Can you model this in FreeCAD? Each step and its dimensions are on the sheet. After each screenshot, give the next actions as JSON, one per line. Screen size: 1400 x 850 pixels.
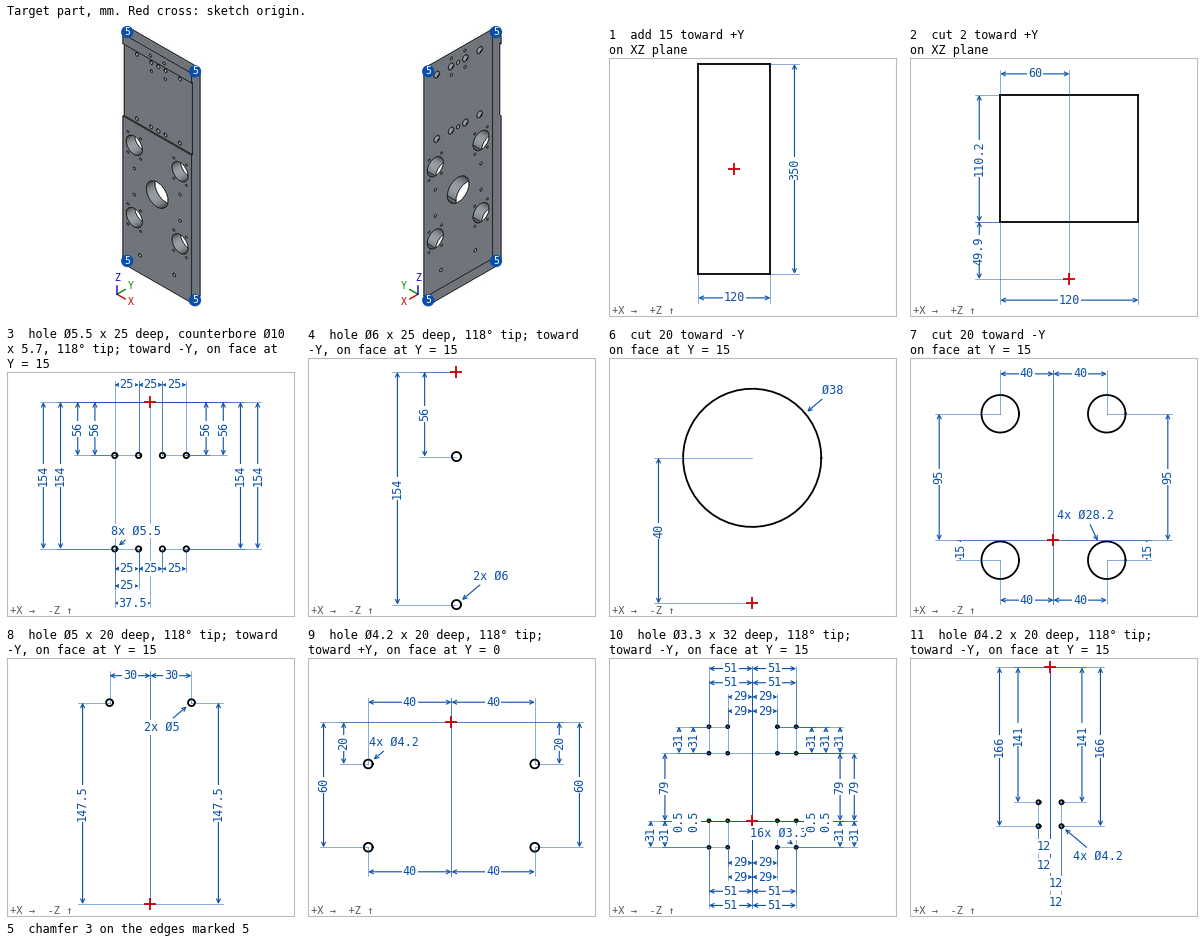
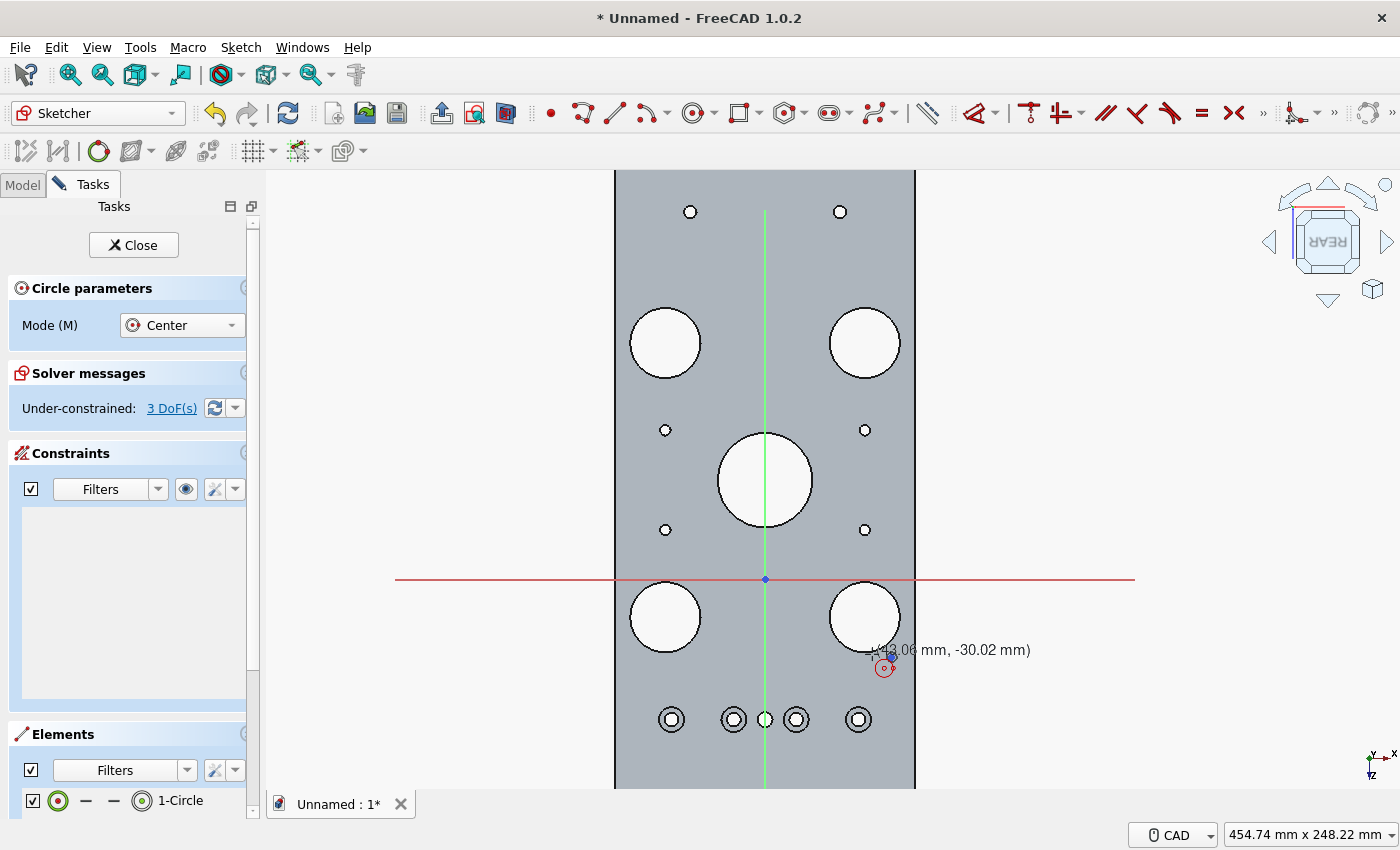
{"action": "left_click", "coordinate": [837, 656]}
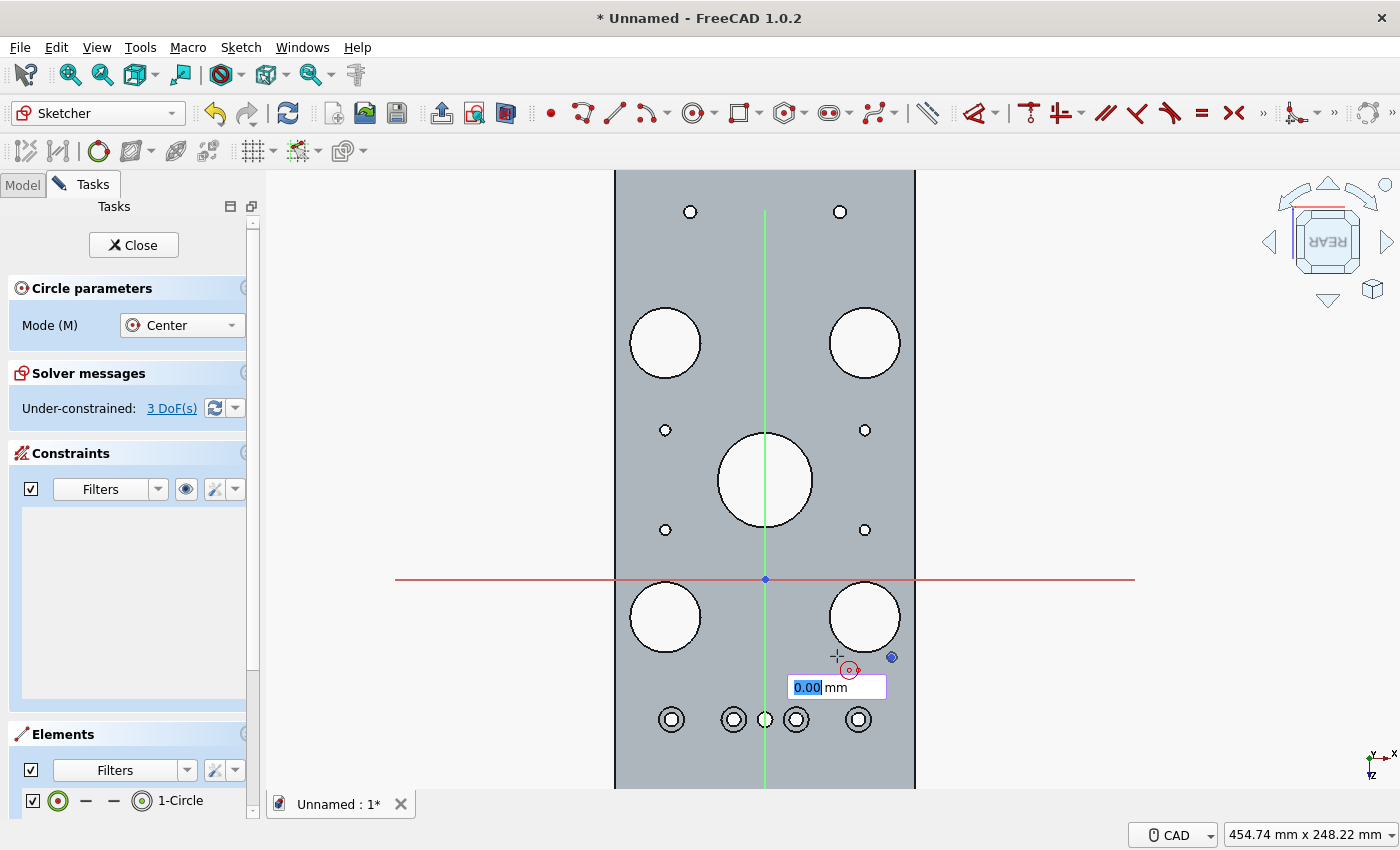
{"action": "scroll", "coordinate": [840, 653], "scroll_direction": "up", "scroll_amount": 7}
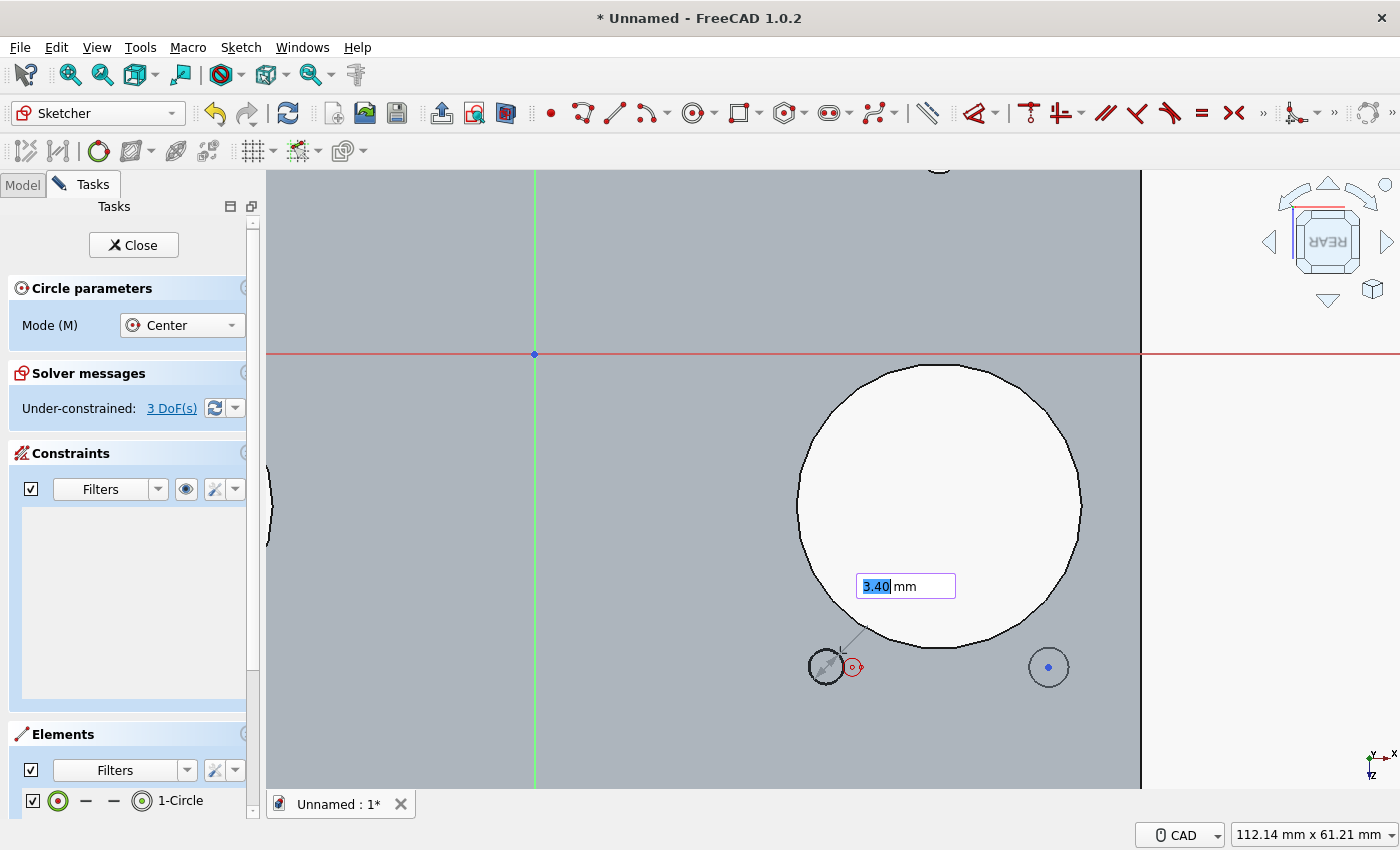
{"action": "left_click", "coordinate": [840, 651]}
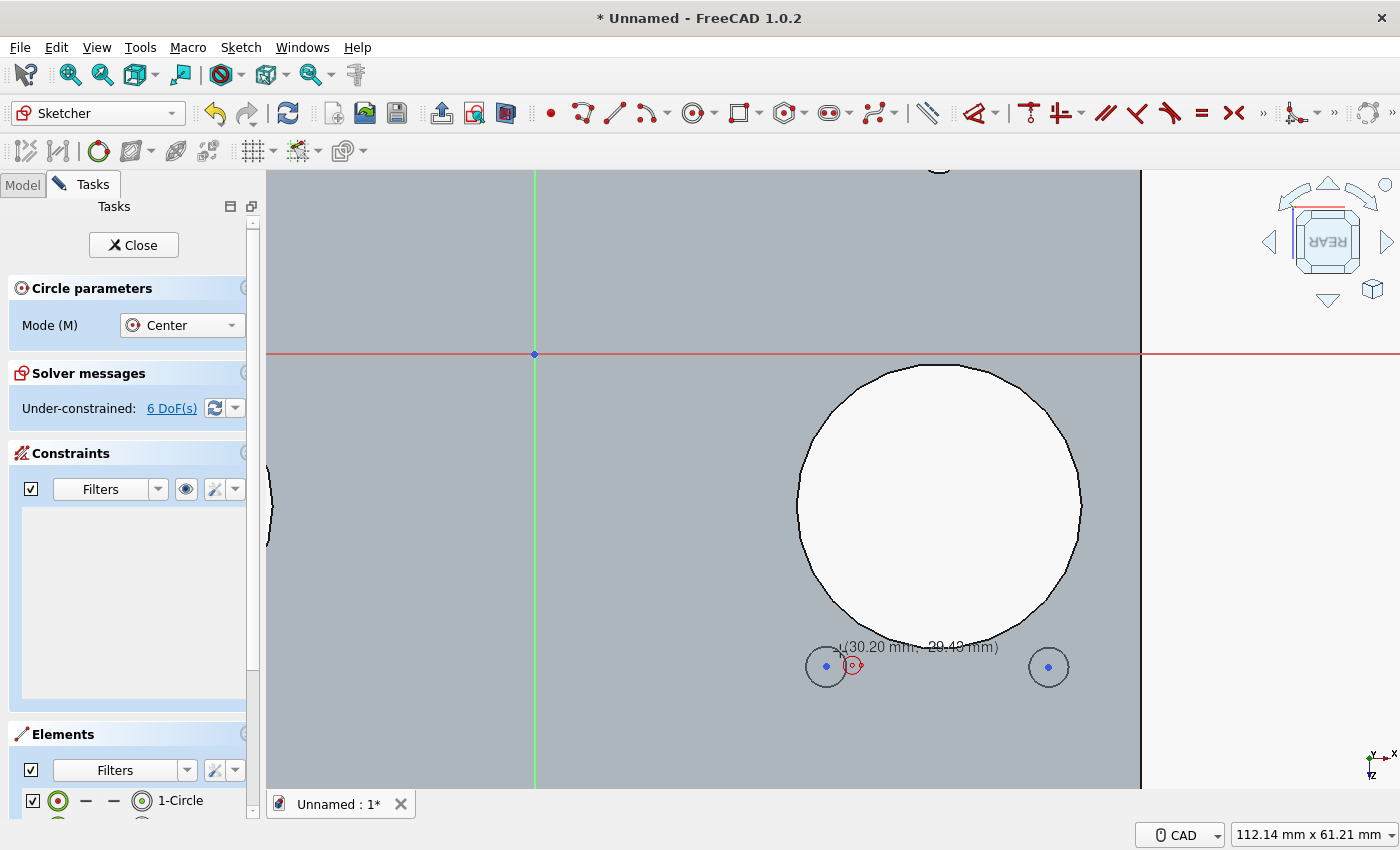
{"action": "scroll", "coordinate": [1050, 349], "scroll_direction": "up", "scroll_amount": 6}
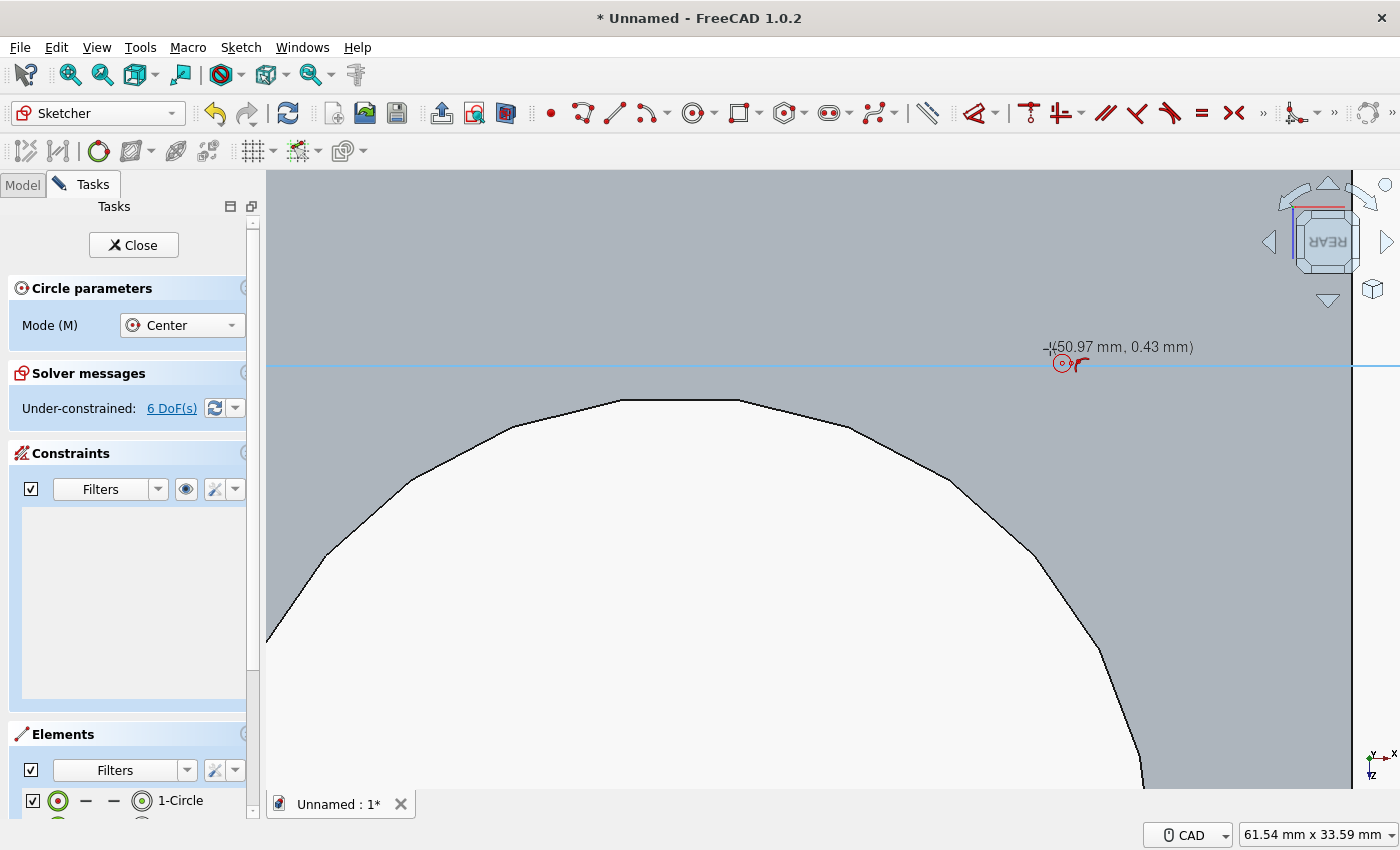
{"action": "left_click", "coordinate": [1050, 349]}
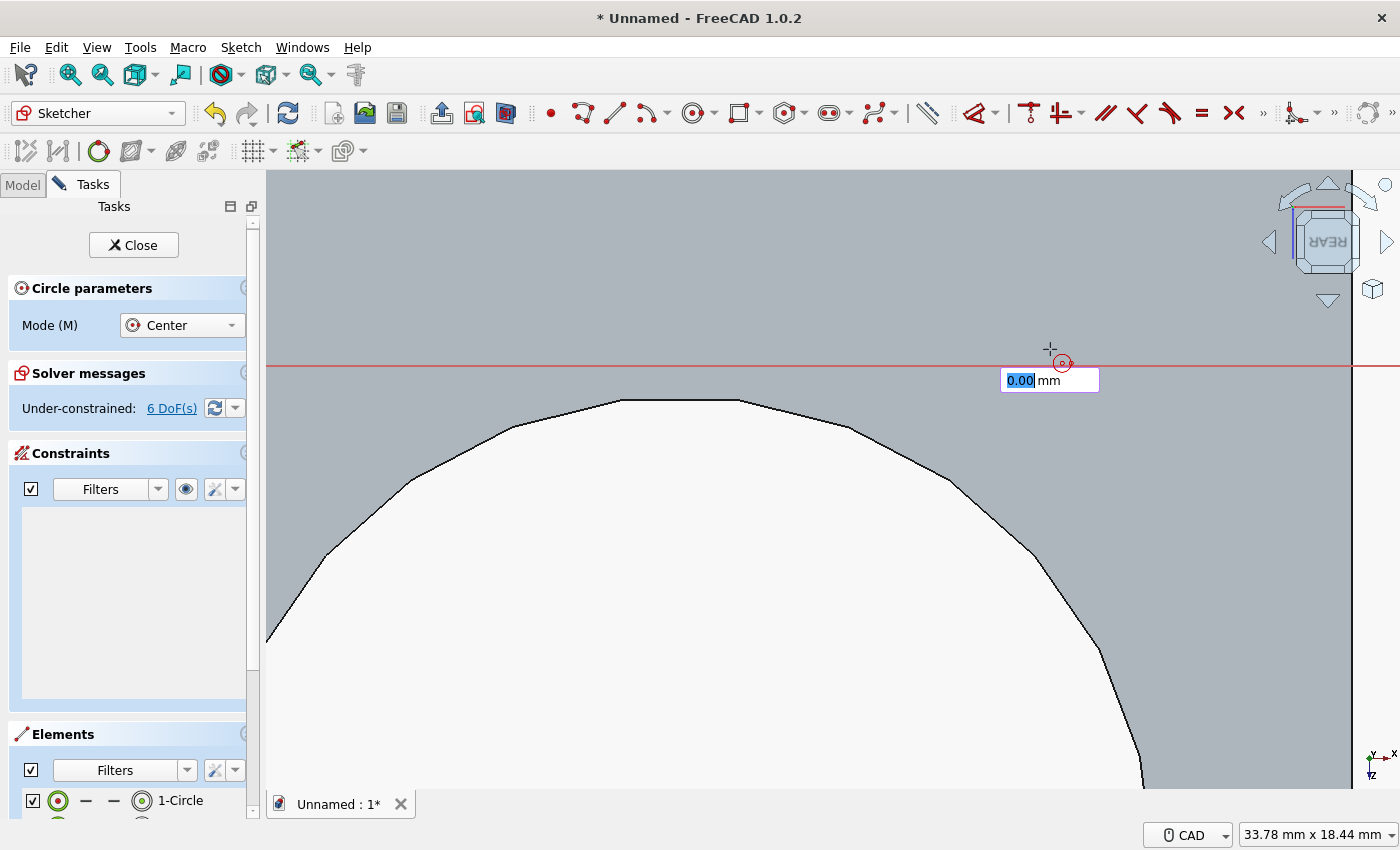
{"action": "scroll", "coordinate": [879, 596], "scroll_direction": "down", "scroll_amount": 13}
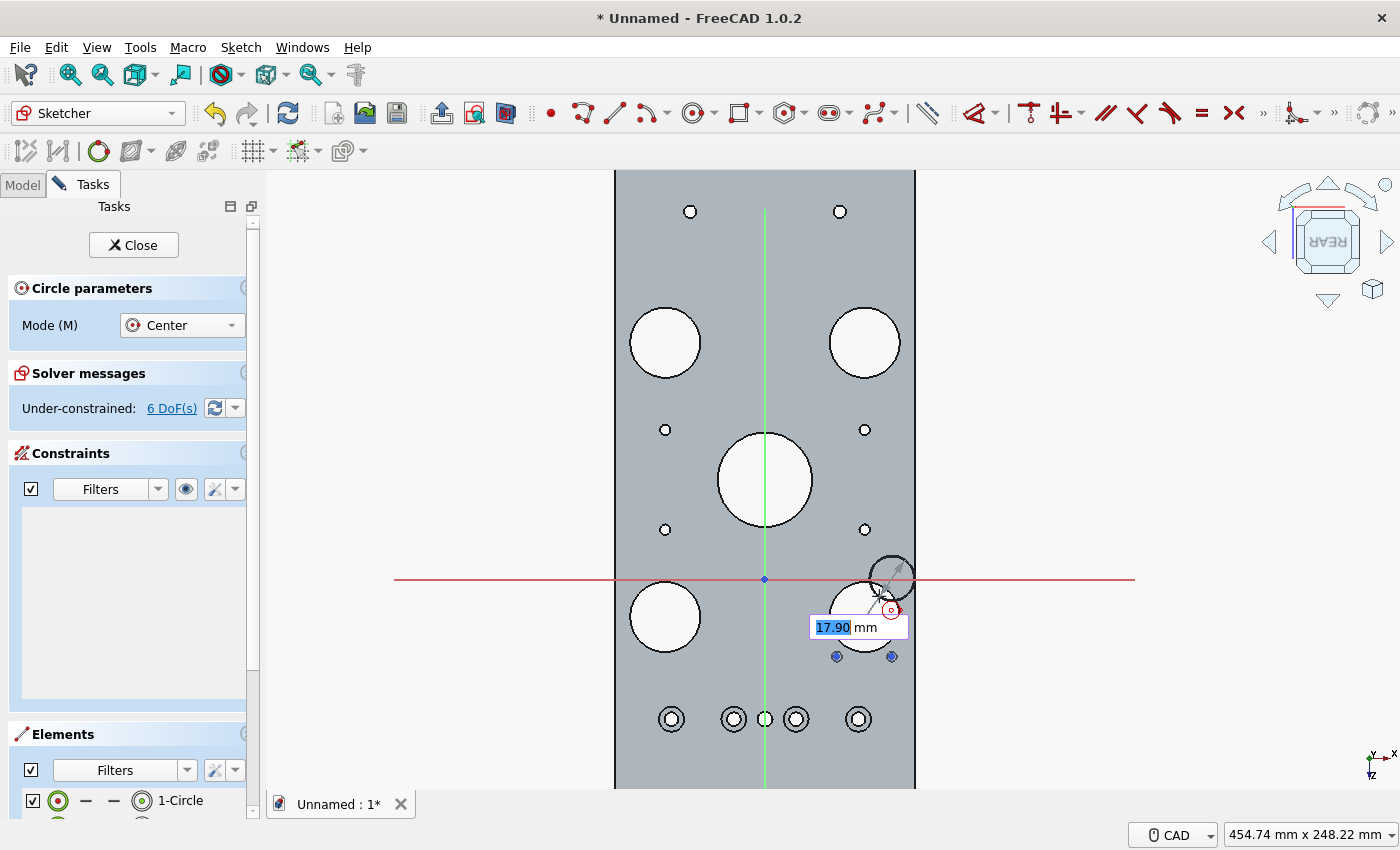
{"action": "scroll", "coordinate": [895, 575], "scroll_direction": "up", "scroll_amount": 7}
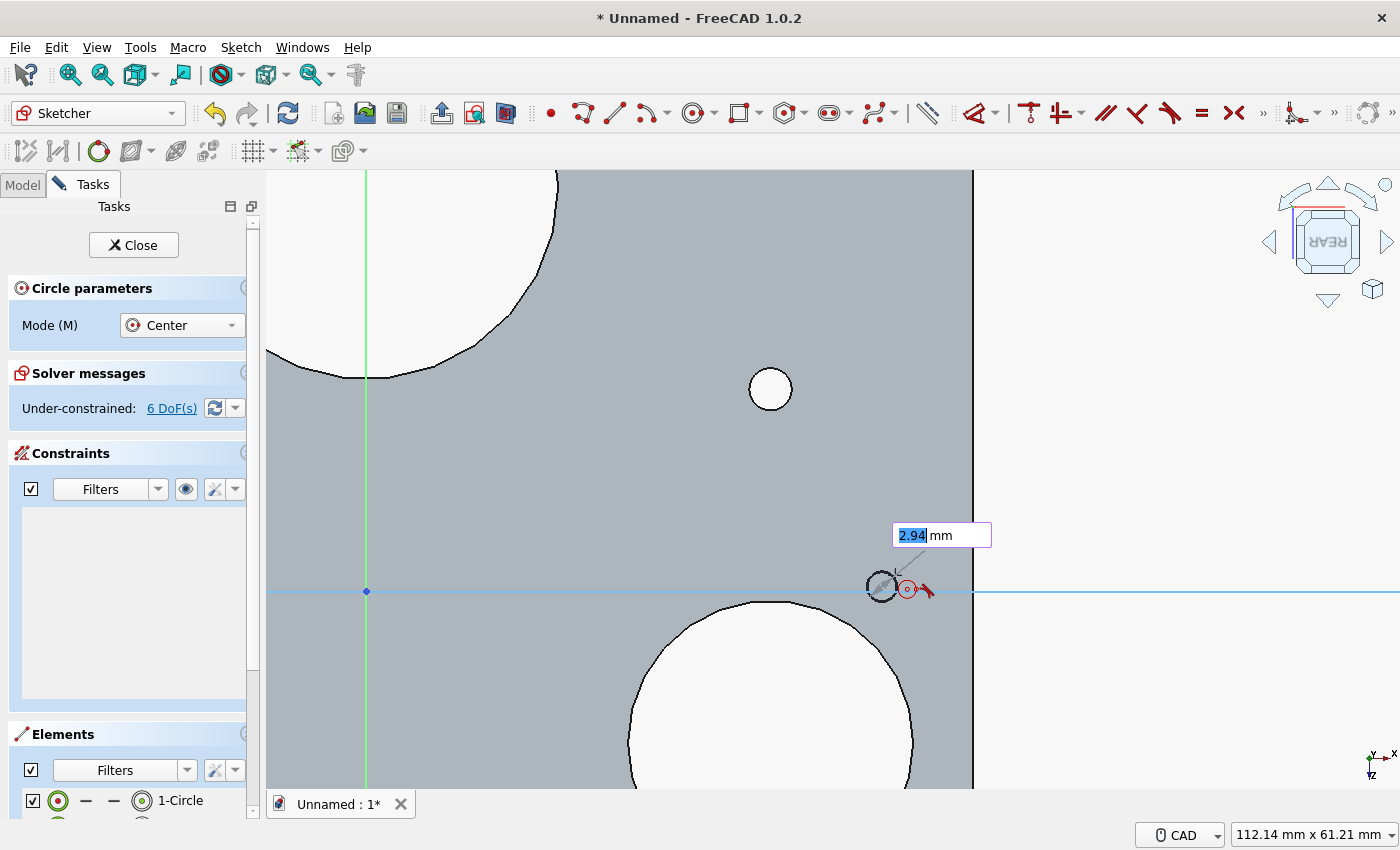
{"action": "left_click", "coordinate": [894, 575]}